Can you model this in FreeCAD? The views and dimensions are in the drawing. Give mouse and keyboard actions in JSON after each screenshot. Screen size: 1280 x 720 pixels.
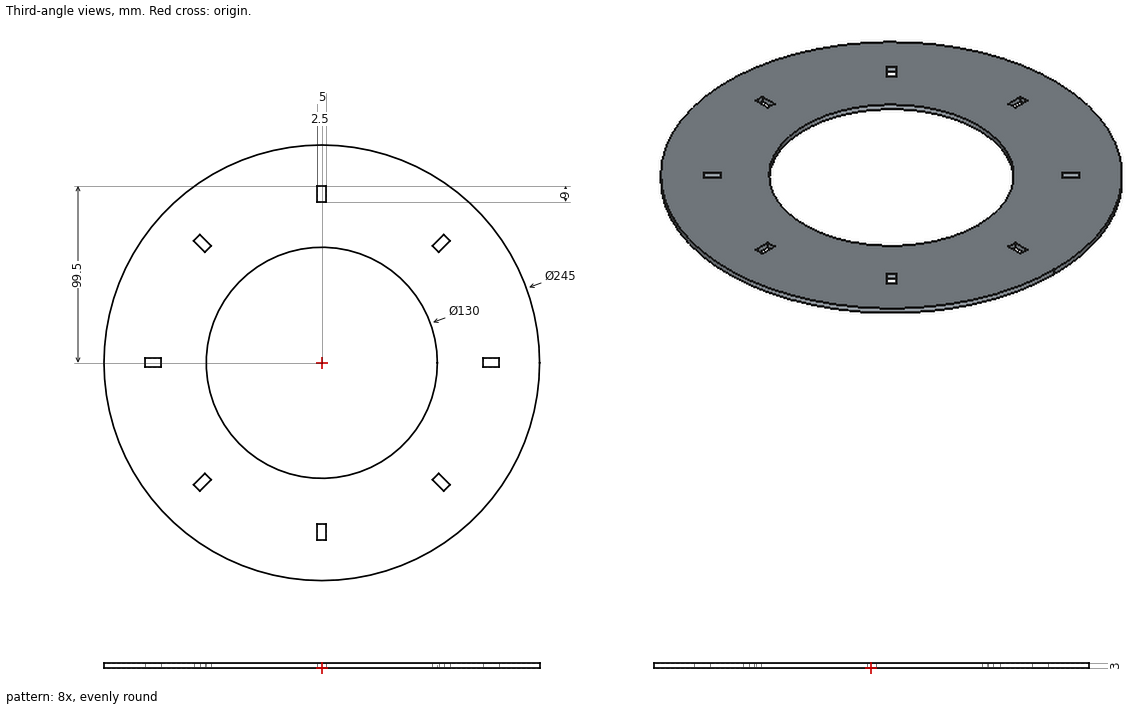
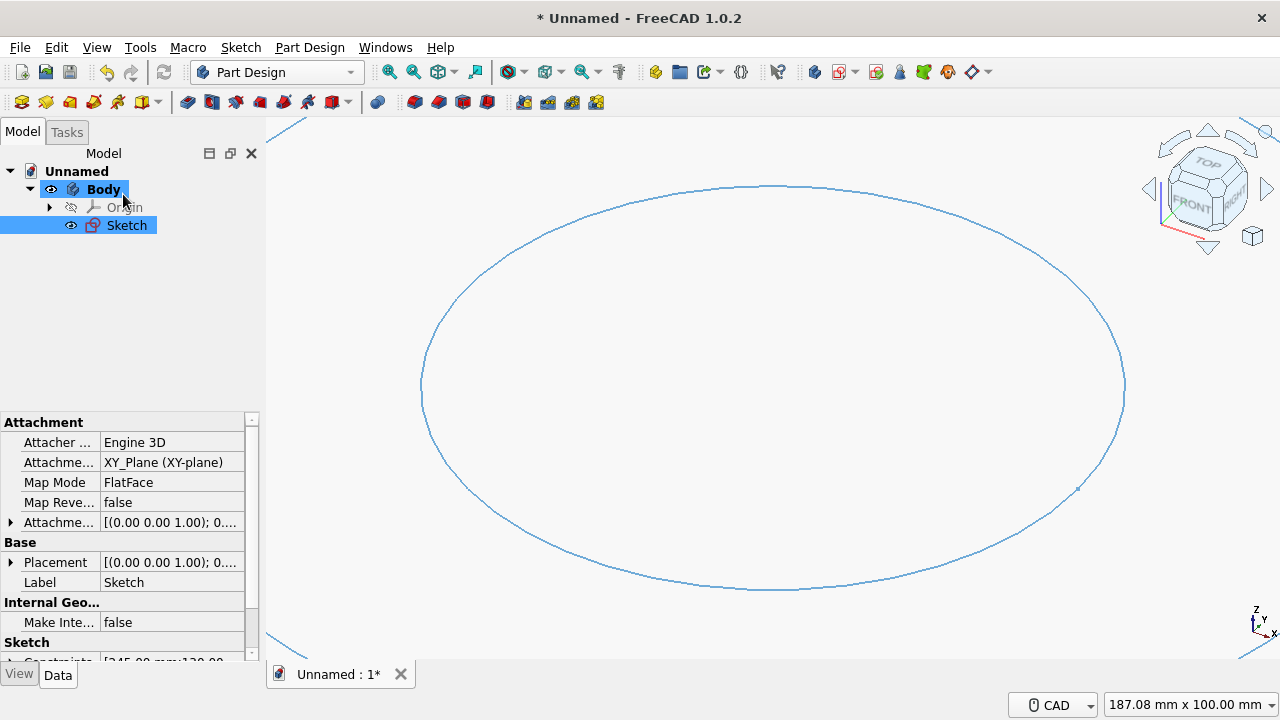
{"action": "left_click", "coordinate": [22, 102]}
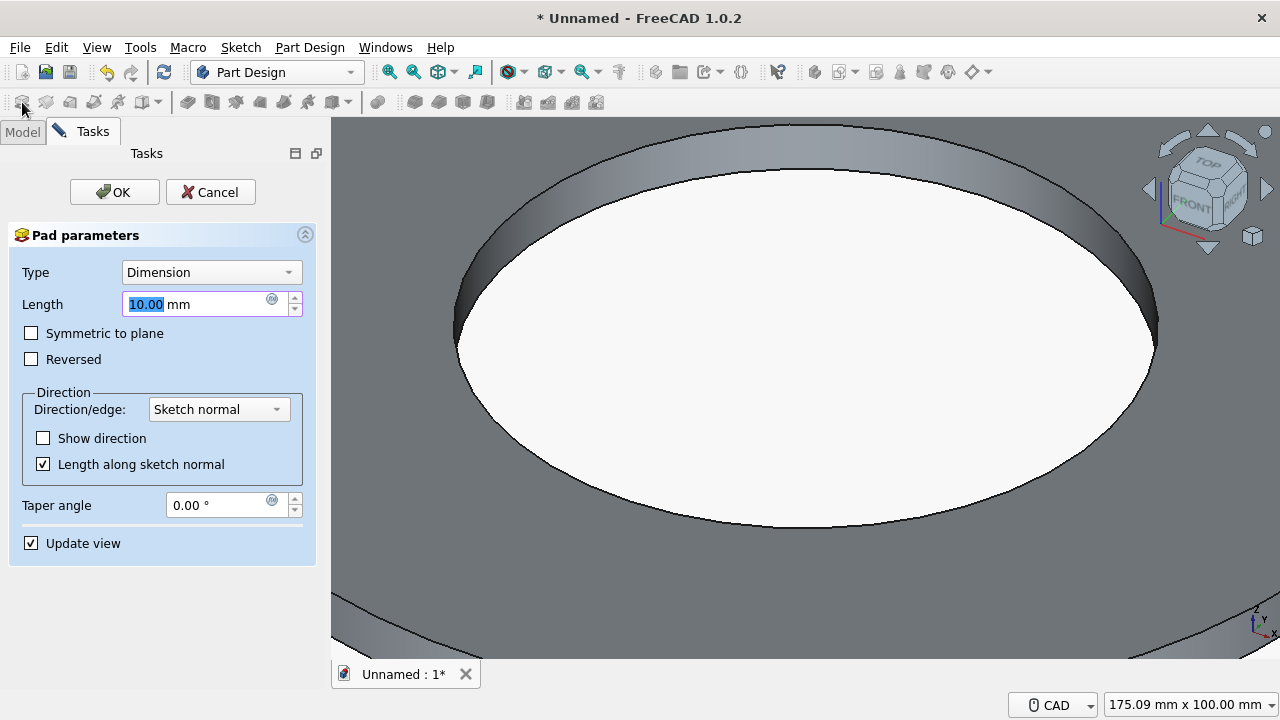
{"action": "type", "text": "3"}
{"action": "key", "text": "Tab"}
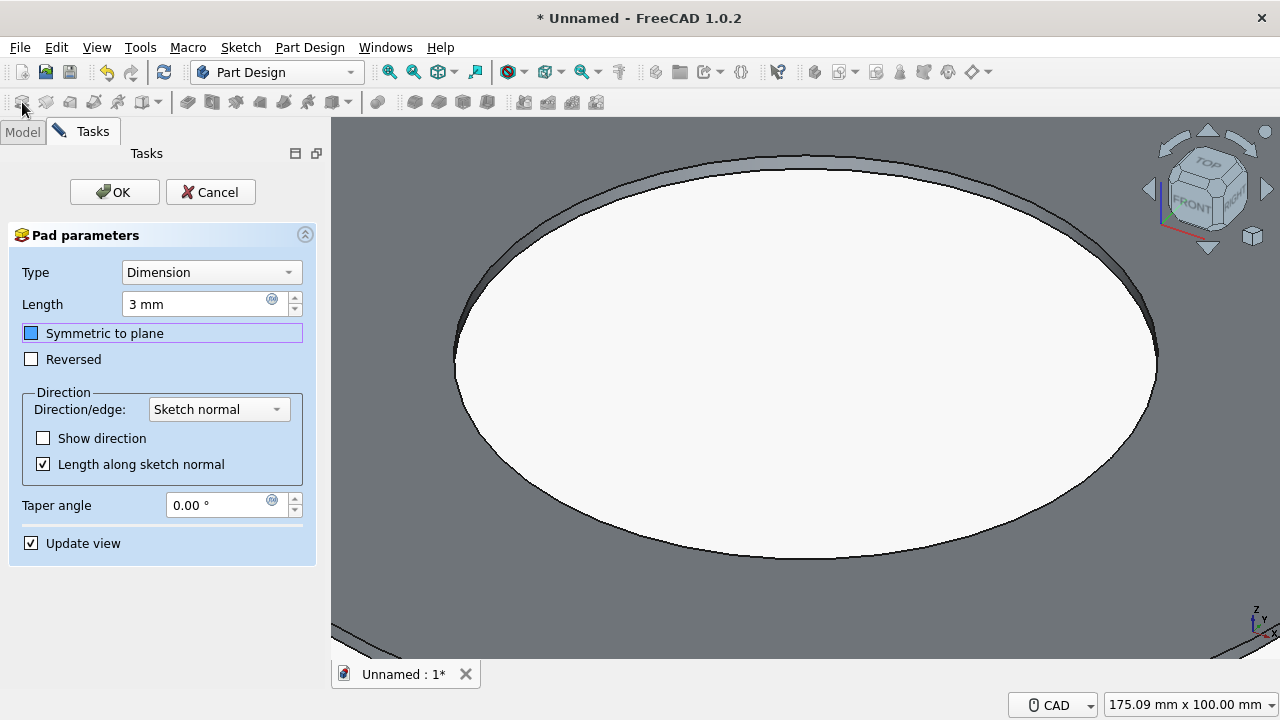
{"action": "left_click", "coordinate": [115, 192]}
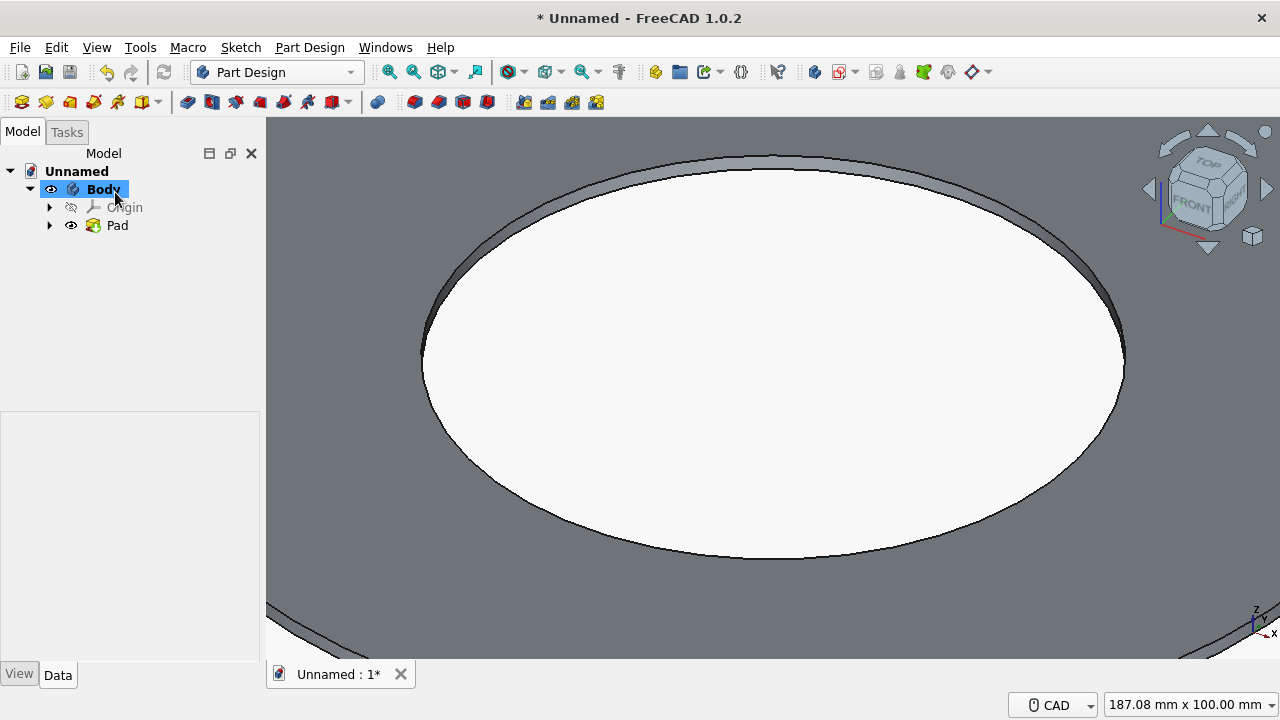
{"action": "key", "text": "v f"}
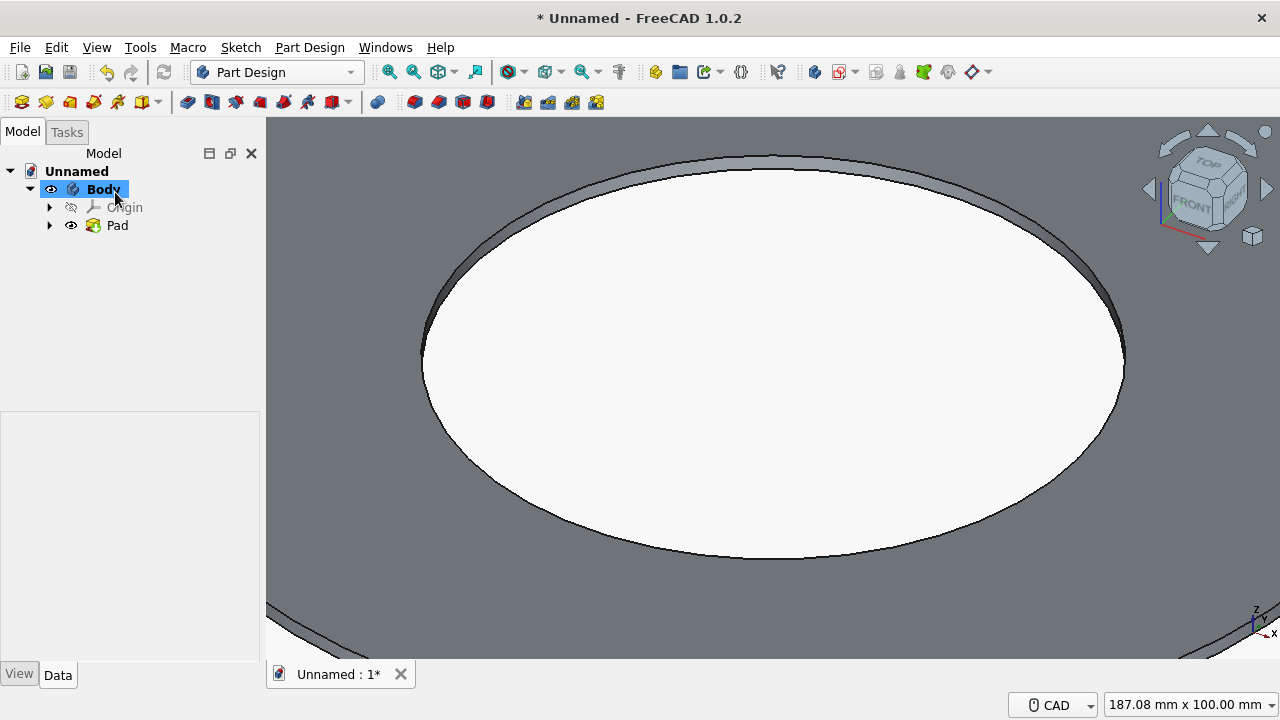
{"action": "left_click", "coordinate": [623, 408]}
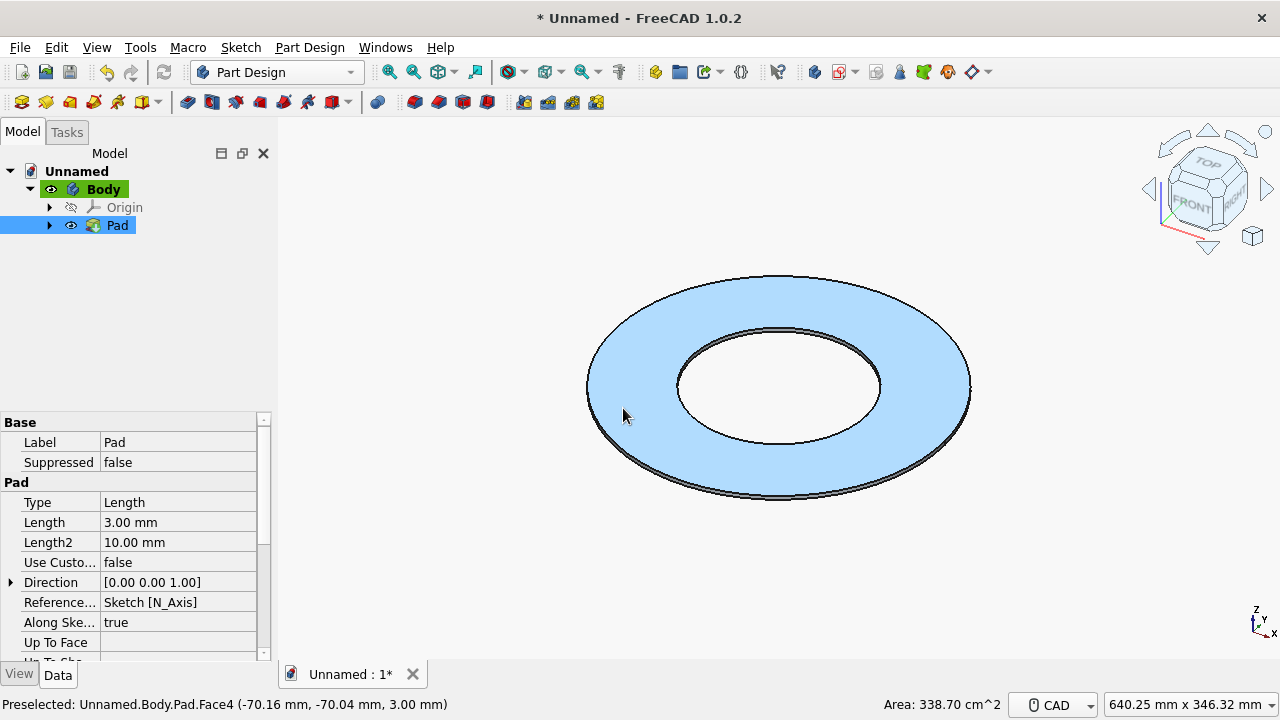
{"action": "left_click", "coordinate": [840, 72]}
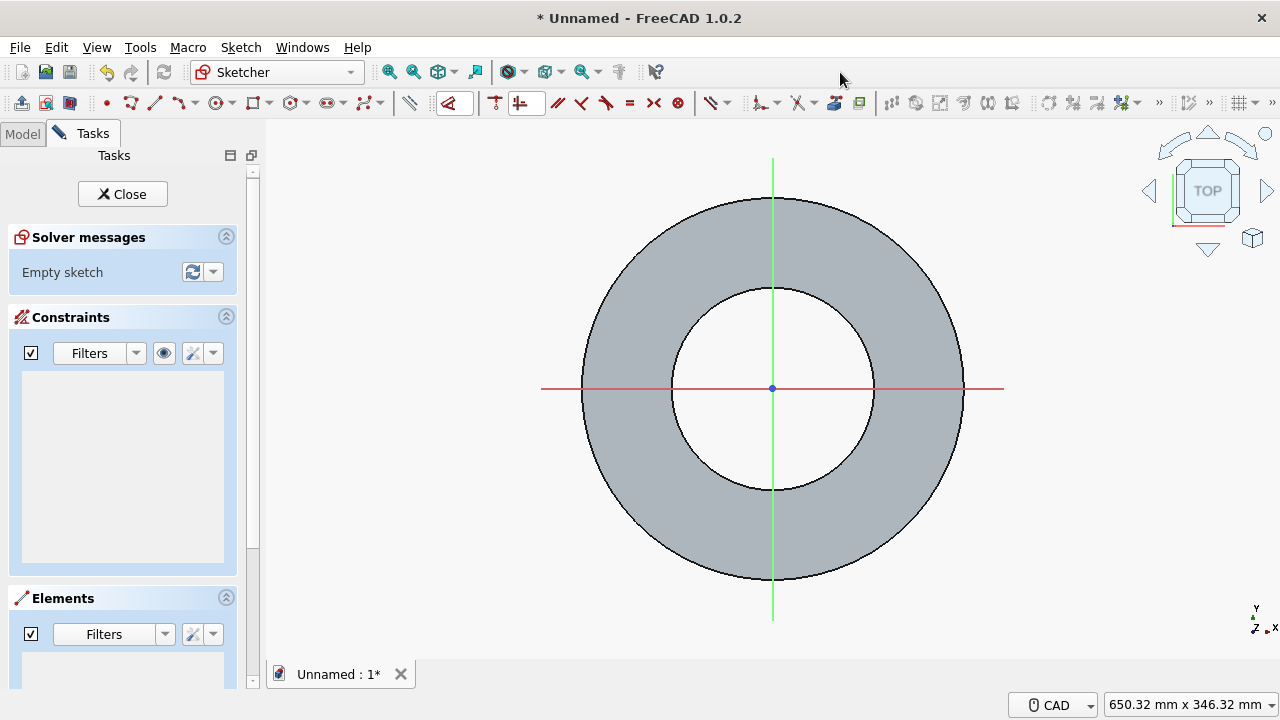
{"action": "scroll", "coordinate": [776, 233], "scroll_direction": "up", "scroll_amount": 15}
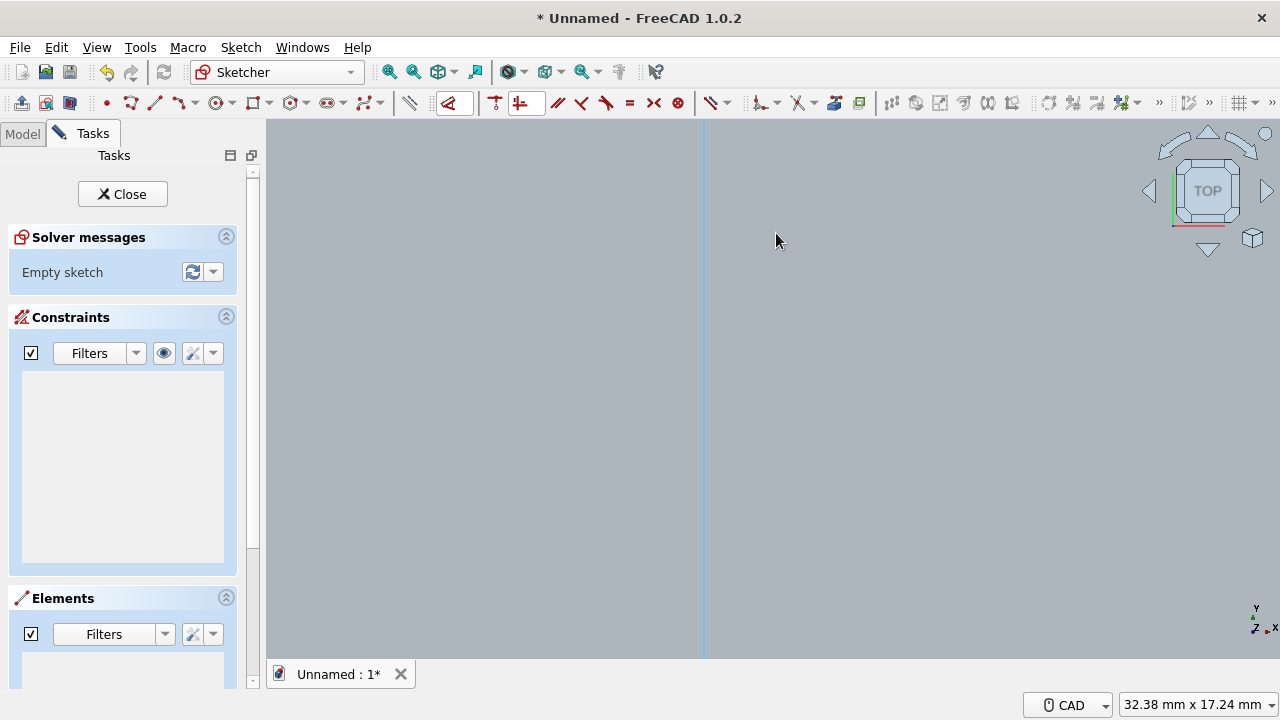
{"action": "left_click", "coordinate": [254, 104]}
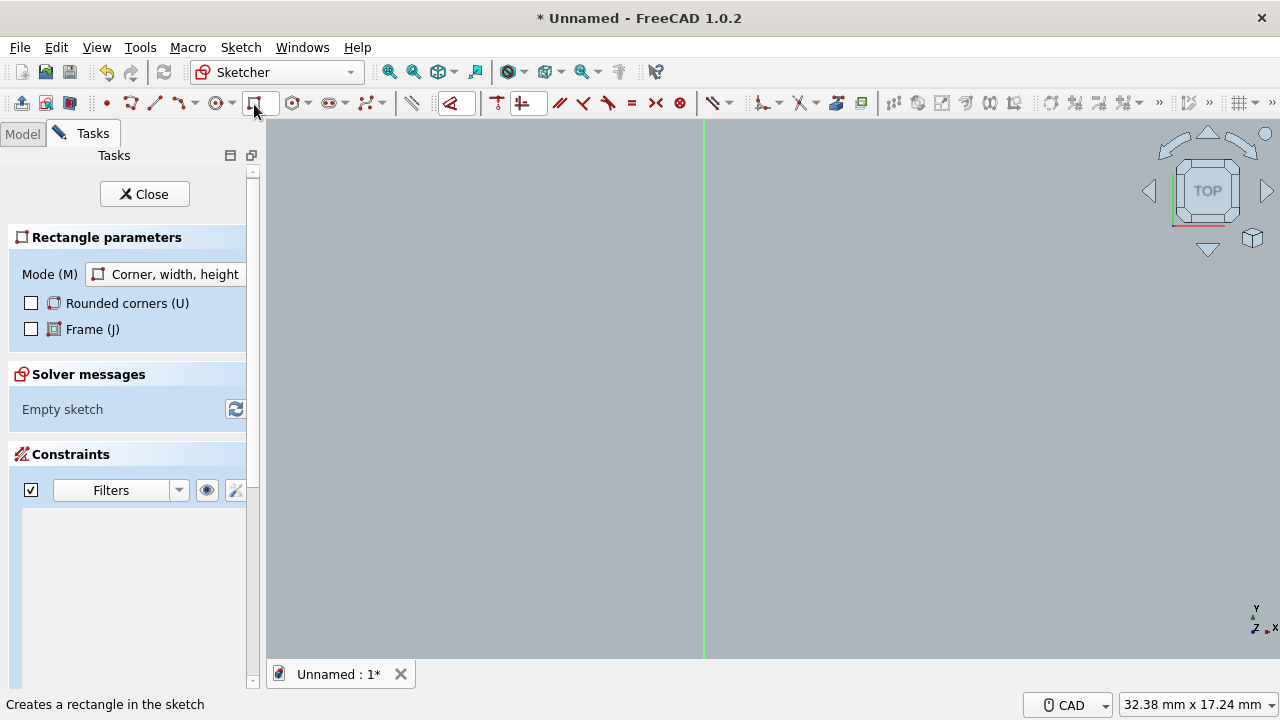
{"action": "left_click", "coordinate": [625, 246]}
{"action": "mouse_move", "coordinate": [782, 528]}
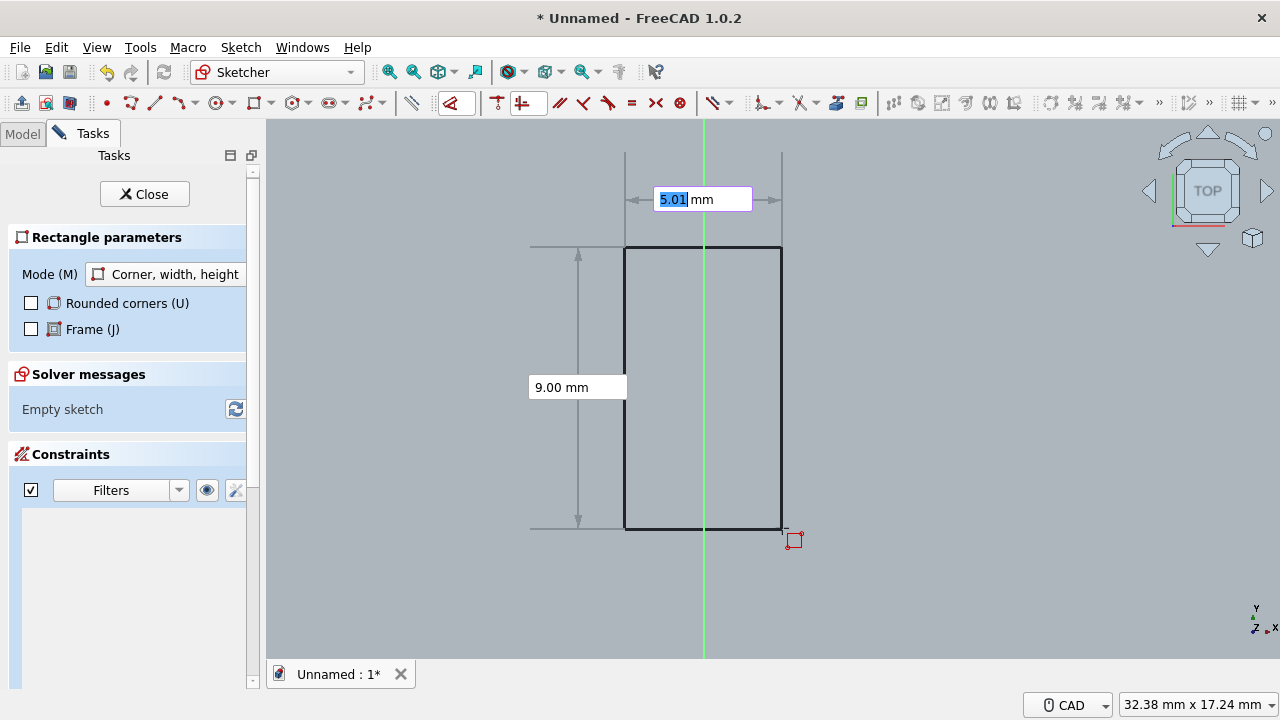
{"action": "type", "text": "5"}
{"action": "key", "text": "Tab"}
{"action": "type", "text": "9"}
{"action": "key", "text": "Return"}
{"action": "key", "text": "Escape"}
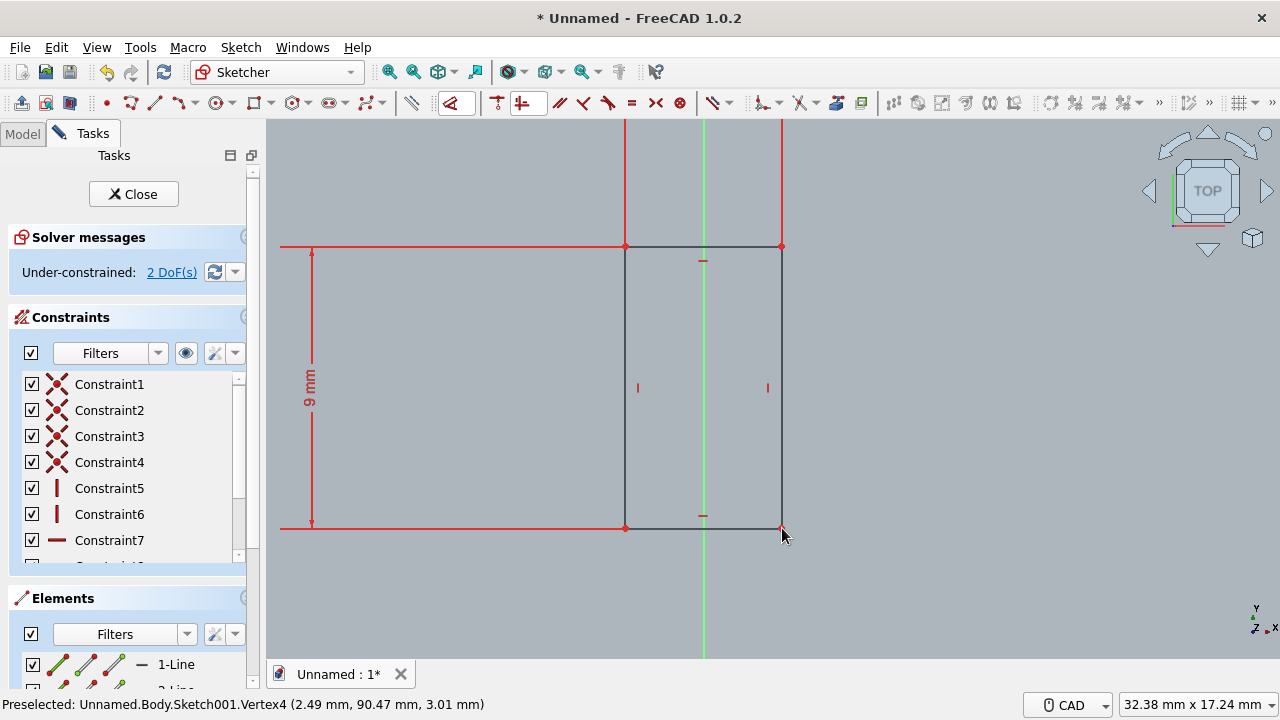
{"action": "key", "text": "d"}